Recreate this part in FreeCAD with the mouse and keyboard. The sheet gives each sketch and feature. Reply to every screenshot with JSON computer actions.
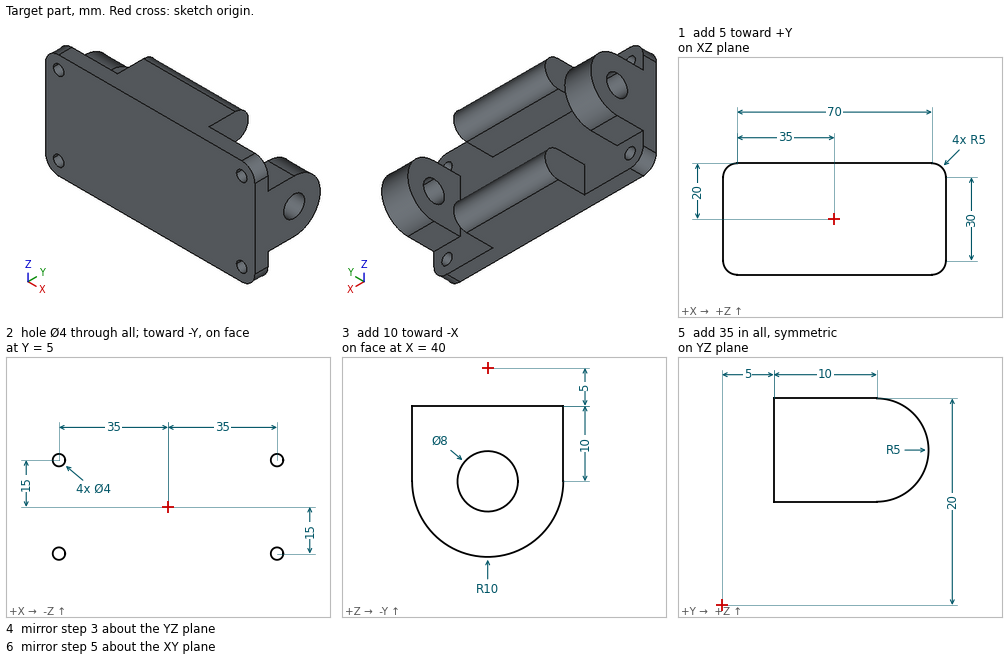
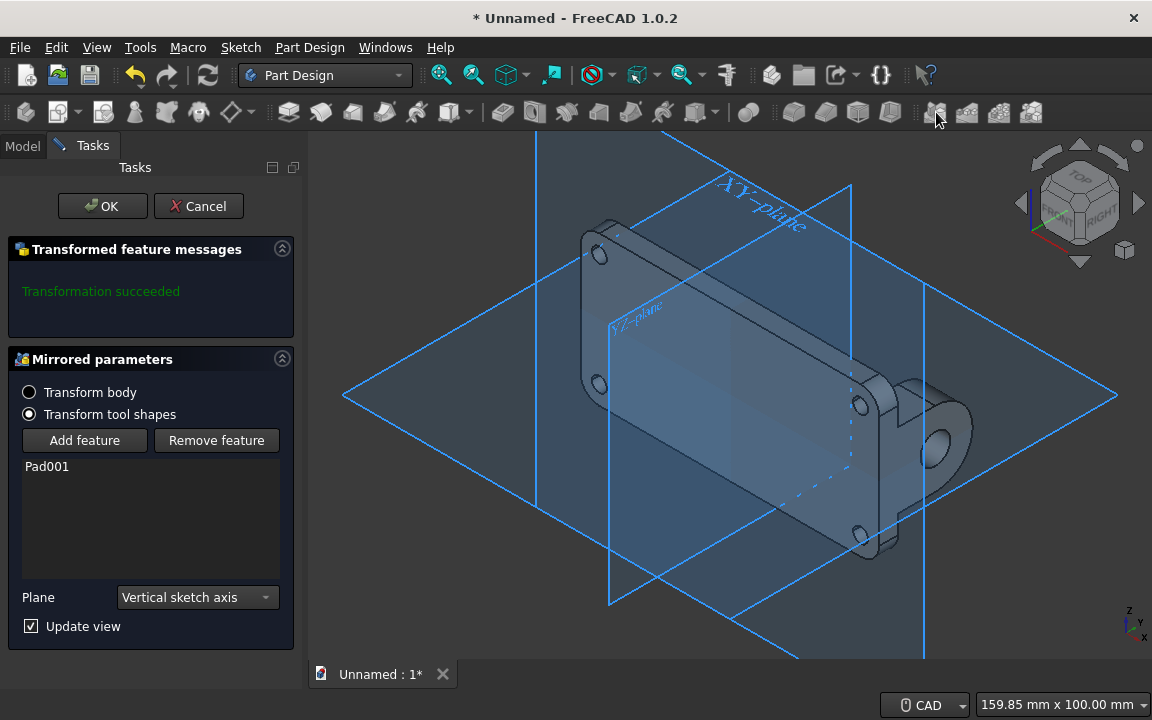
{"action": "left_click", "coordinate": [198, 598]}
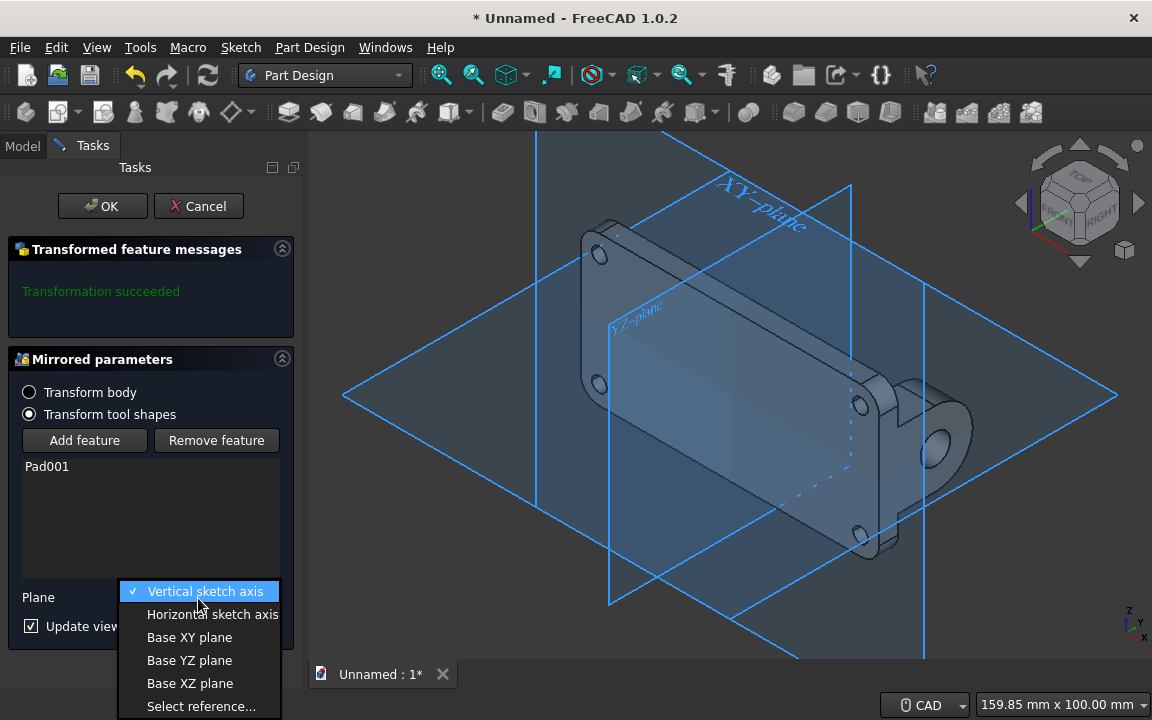
{"action": "left_click", "coordinate": [198, 660]}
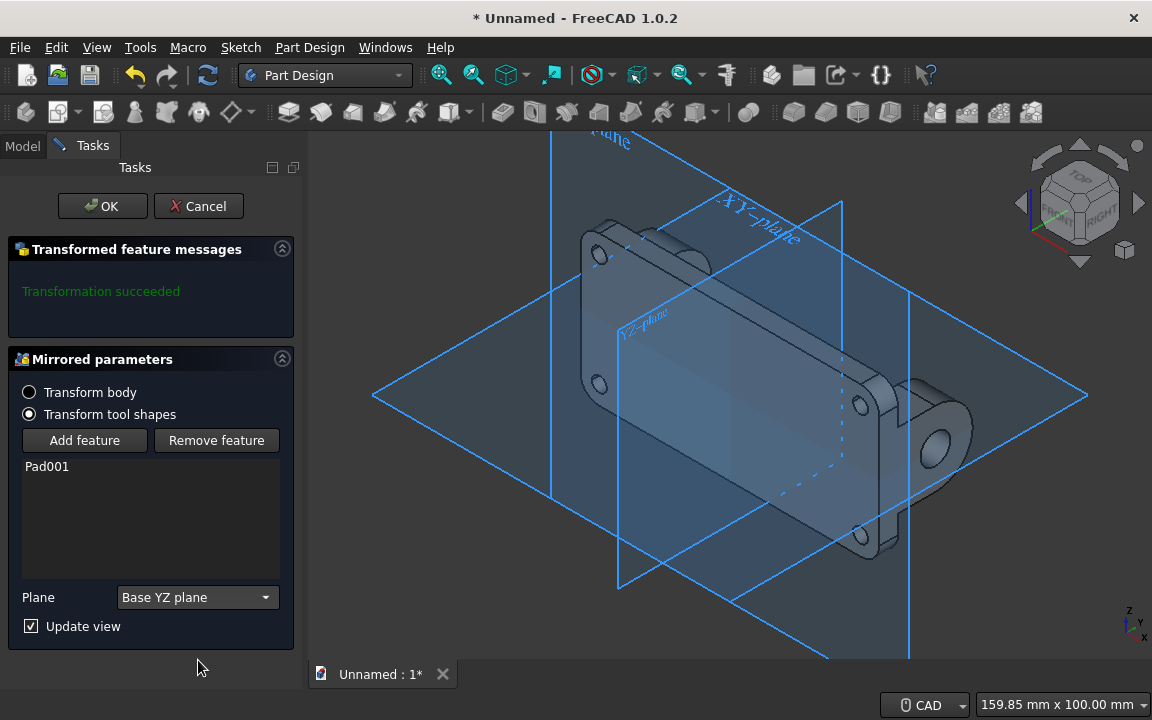
{"action": "left_click", "coordinate": [103, 206]}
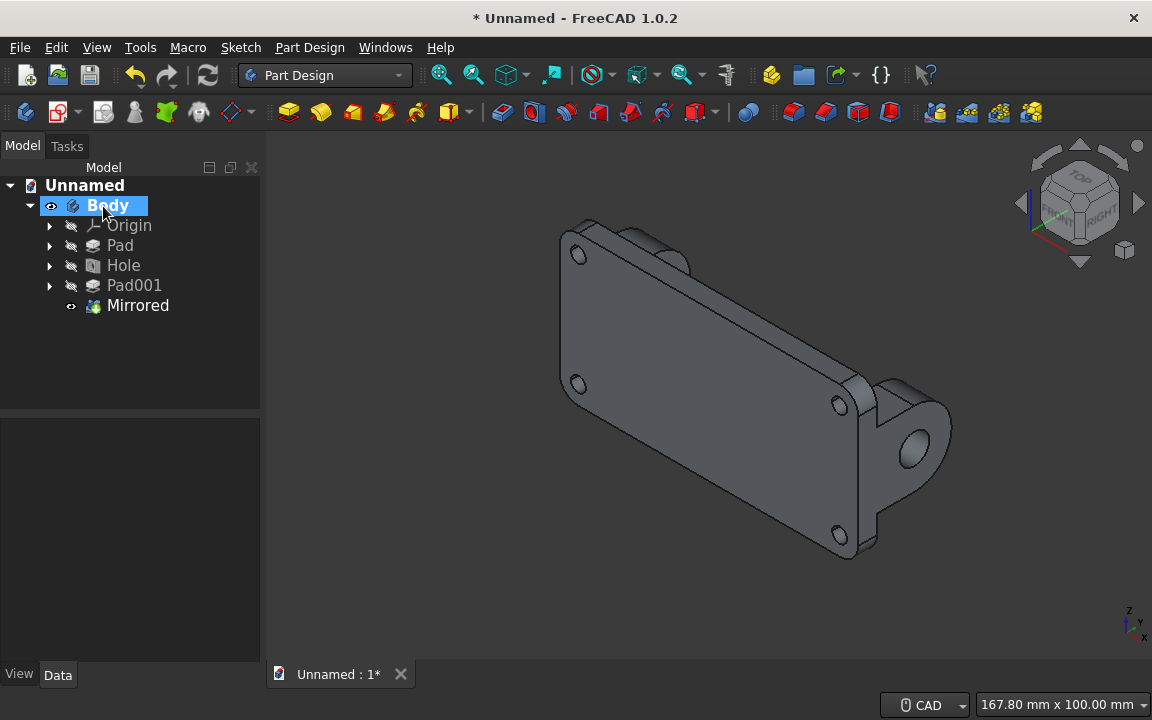
{"action": "left_click", "coordinate": [58, 112]}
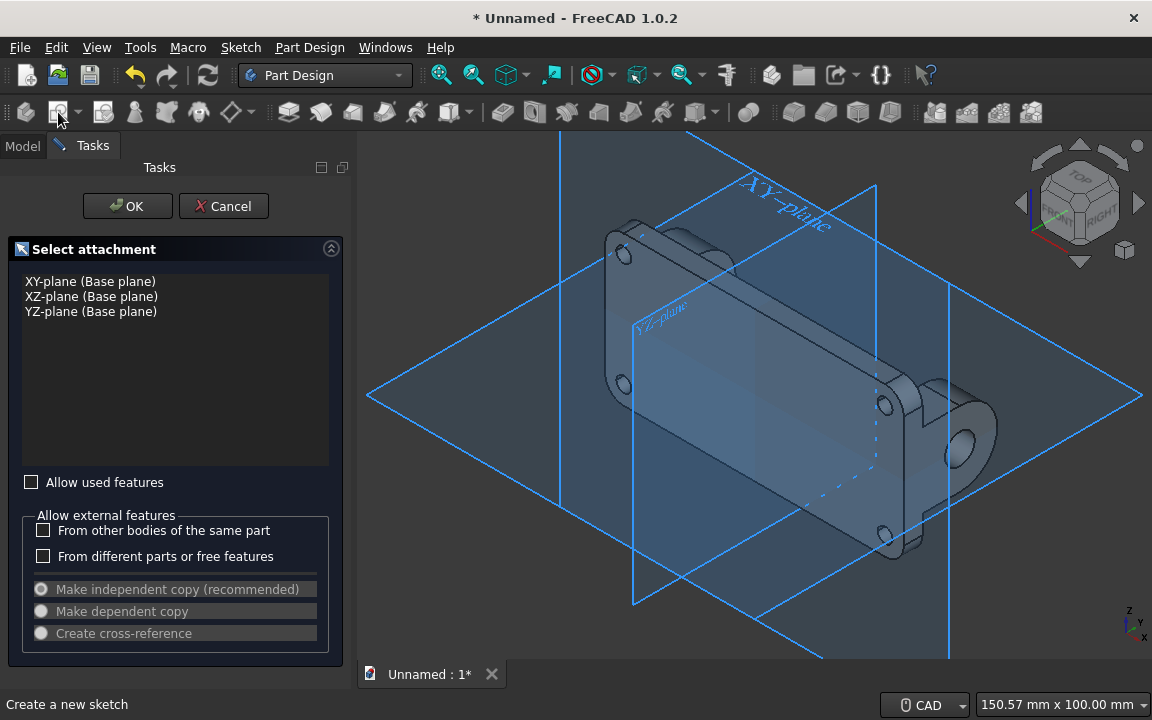
{"action": "left_click", "coordinate": [82, 312]}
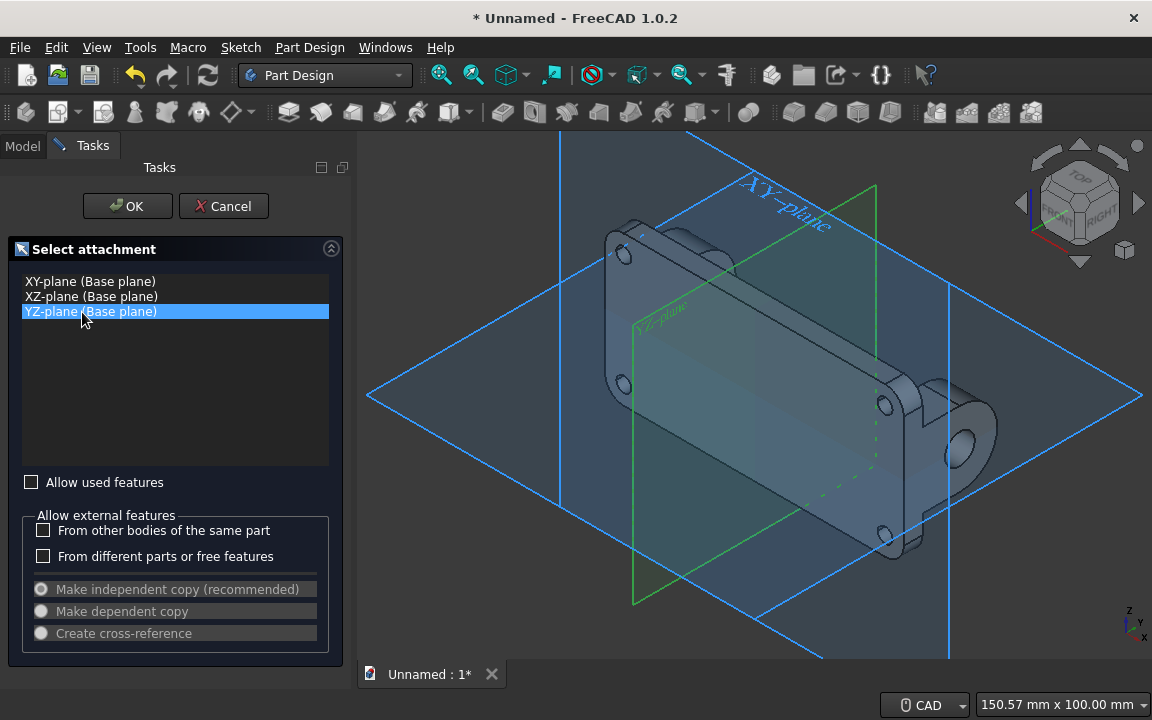
{"action": "left_click", "coordinate": [128, 206]}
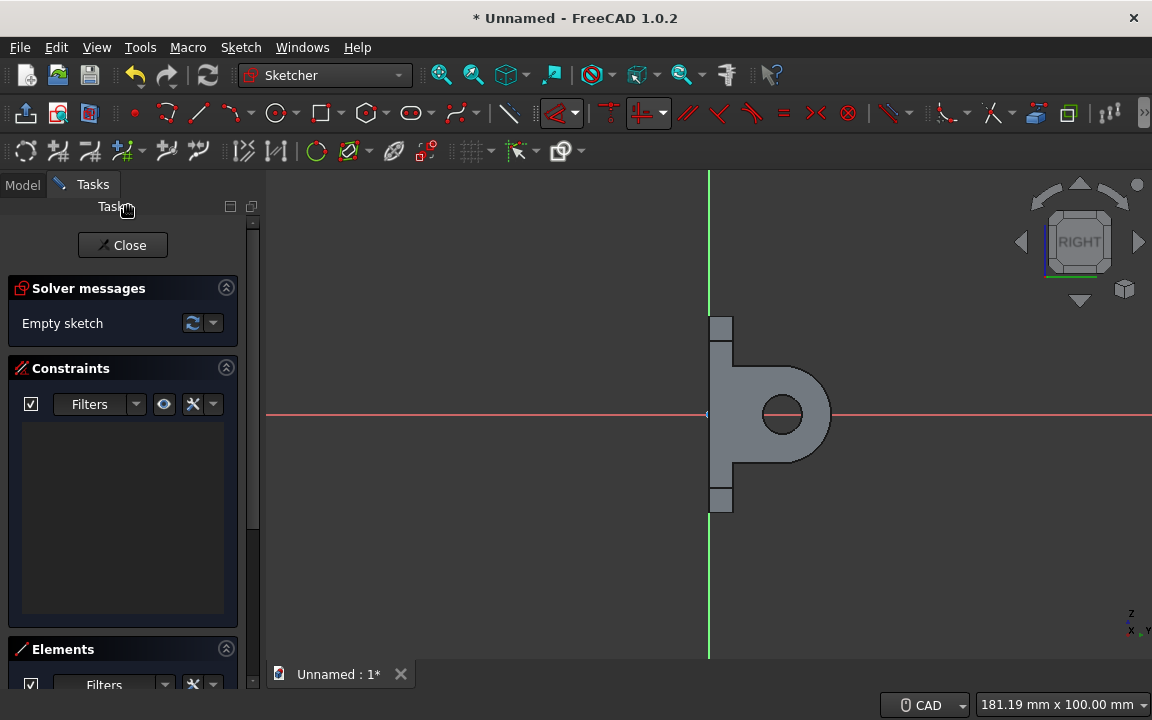
{"action": "left_click", "coordinate": [90, 114]}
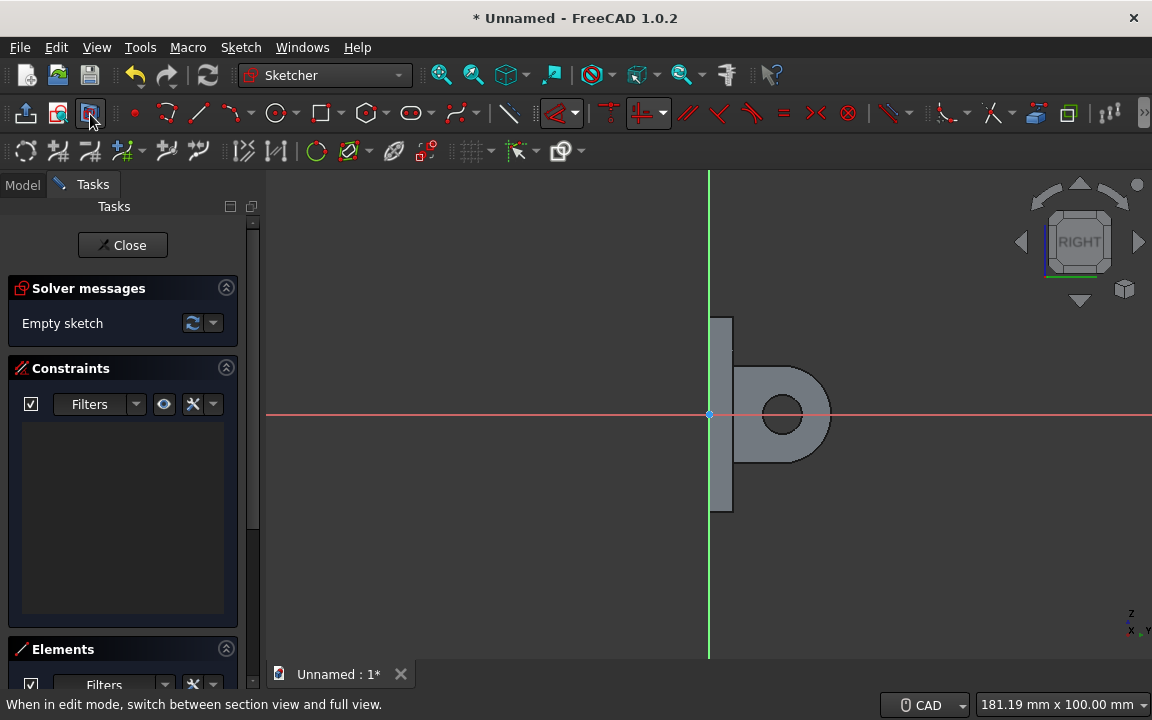
{"action": "scroll", "coordinate": [809, 345], "scroll_direction": "up", "scroll_amount": 6}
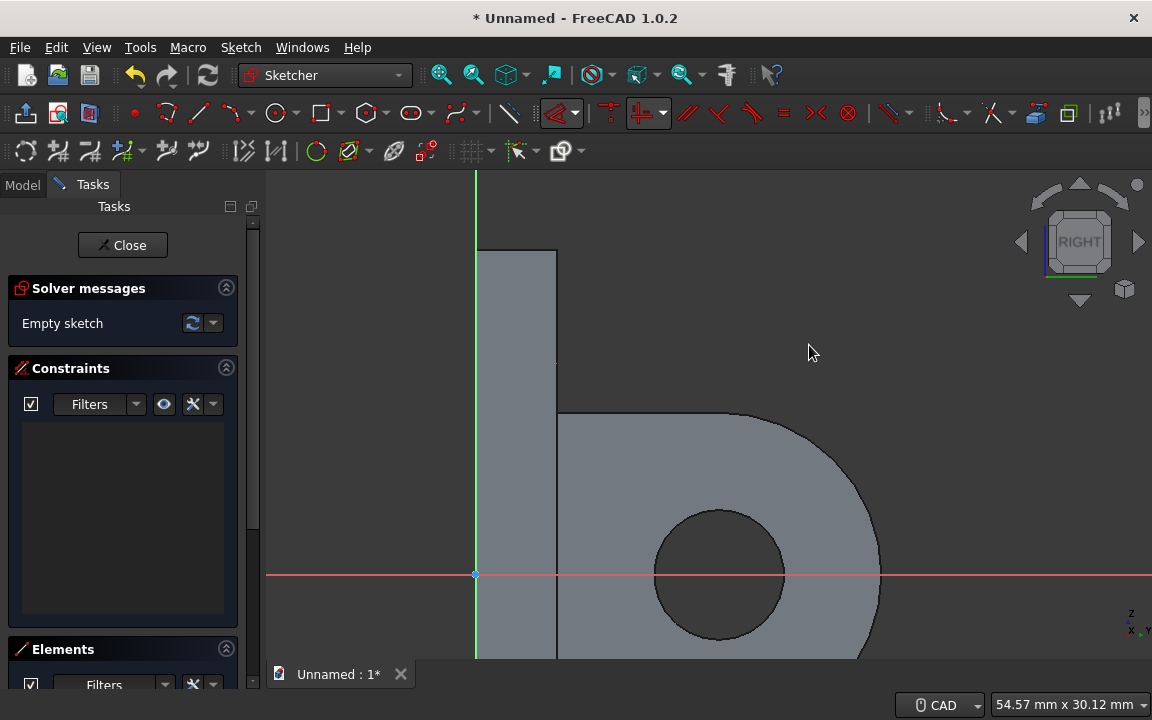
{"action": "key", "text": "g m"}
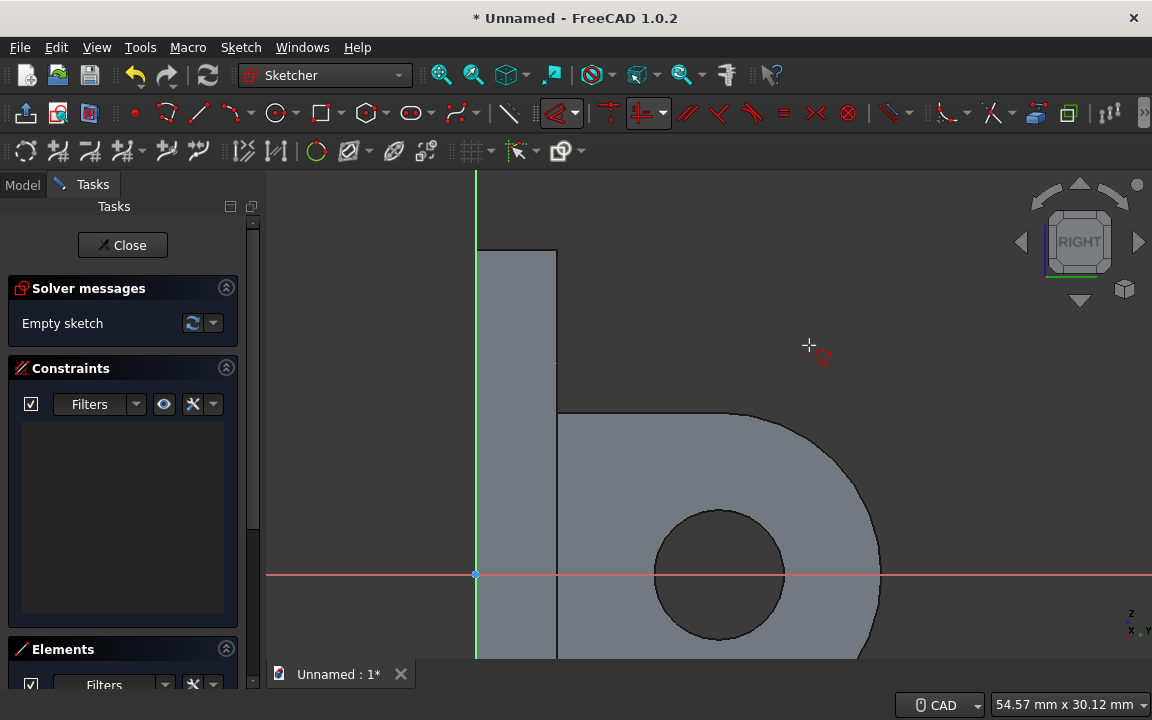
{"action": "left_click", "coordinate": [719, 250]}
{"action": "left_click", "coordinate": [557, 250]}
{"action": "left_click", "coordinate": [557, 413]}
{"action": "left_click", "coordinate": [719, 413]}
{"action": "right_click", "coordinate": [719, 413]}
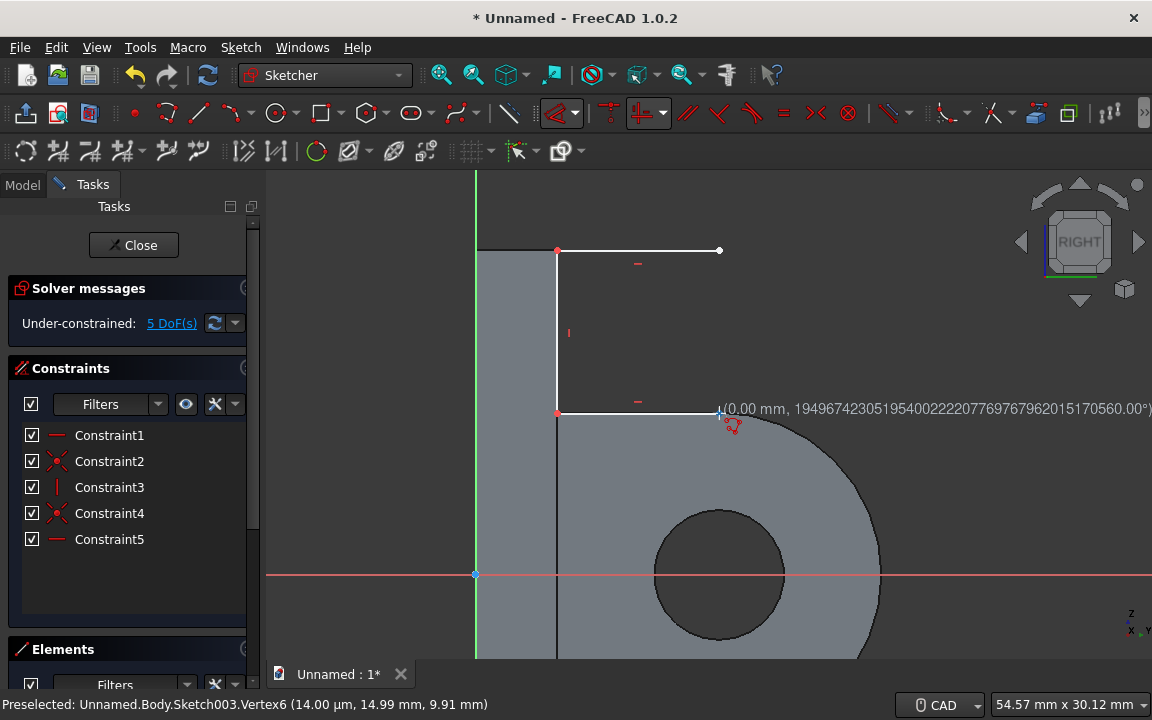
{"action": "key", "text": "g 3 a"}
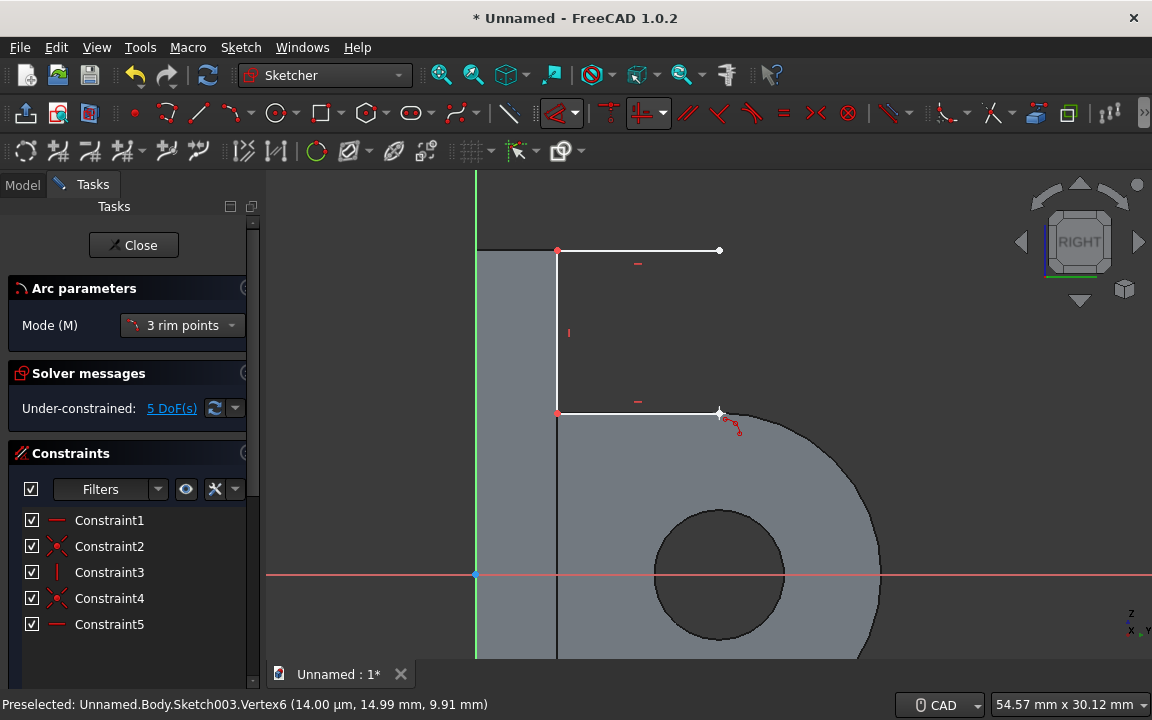
{"action": "left_click", "coordinate": [719, 414]}
{"action": "left_click", "coordinate": [719, 251]}
{"action": "left_click", "coordinate": [800, 331]}
{"action": "key", "text": "Escape"}